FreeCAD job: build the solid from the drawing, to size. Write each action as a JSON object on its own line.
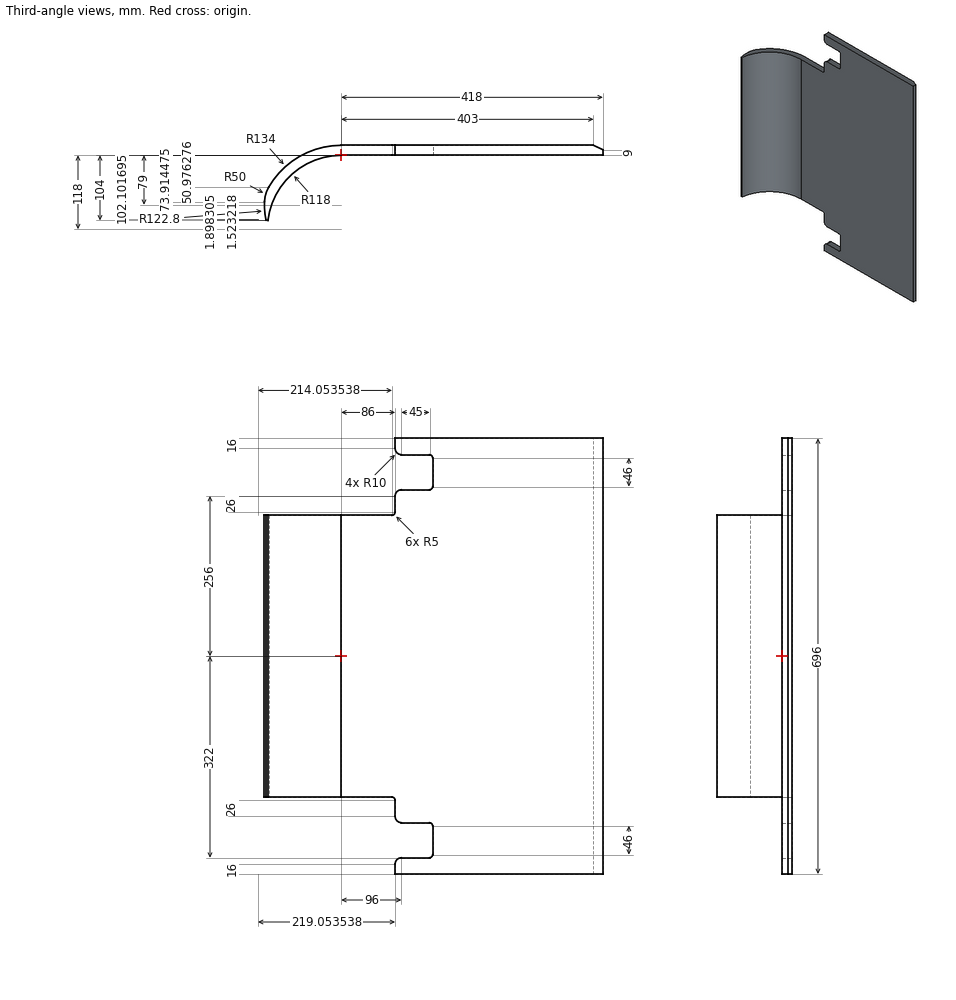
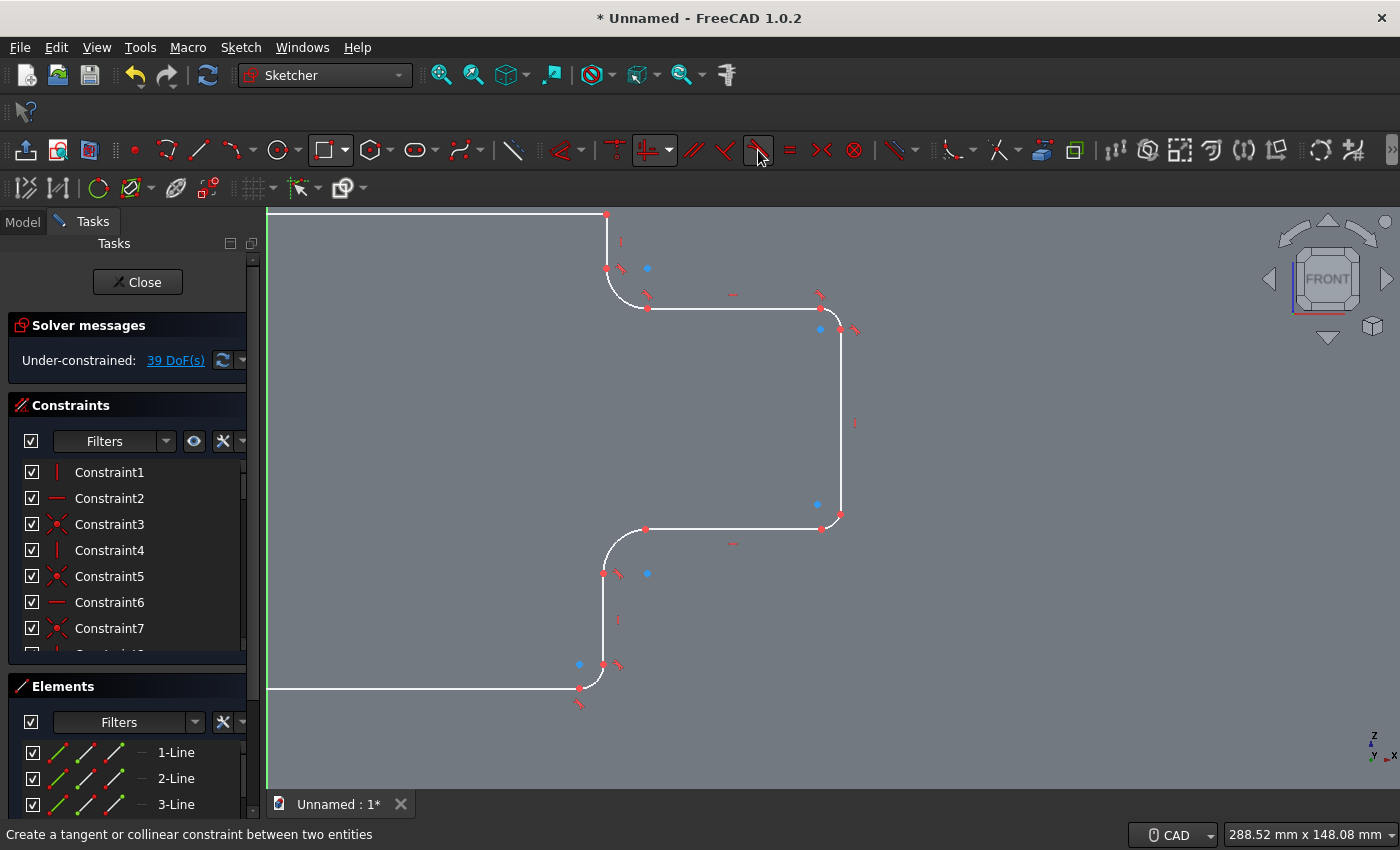
{"action": "scroll", "coordinate": [838, 330], "scroll_direction": "down", "scroll_amount": 10}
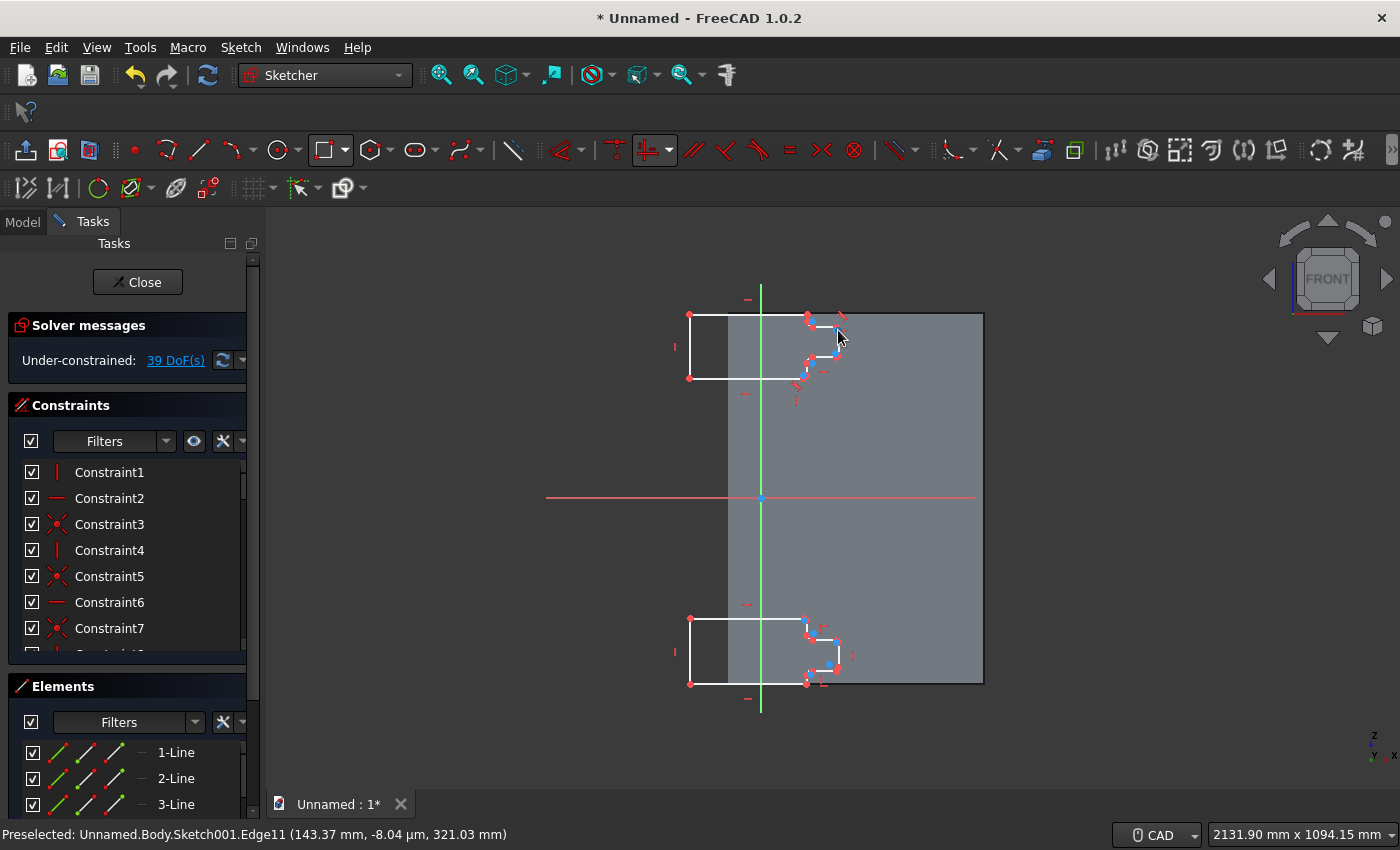
{"action": "scroll", "coordinate": [839, 338], "scroll_direction": "up", "scroll_amount": 4}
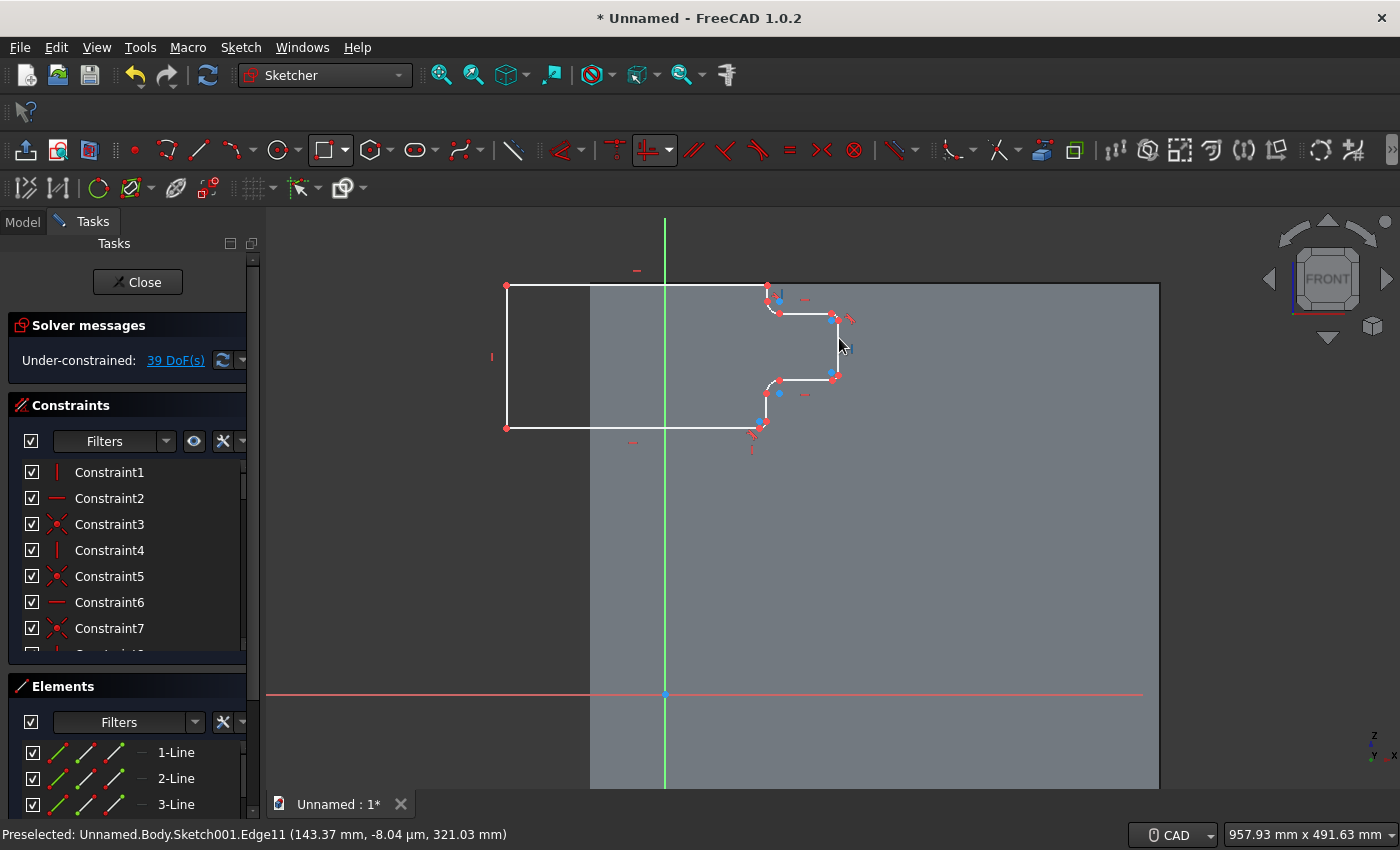
{"action": "left_click", "coordinate": [838, 337]}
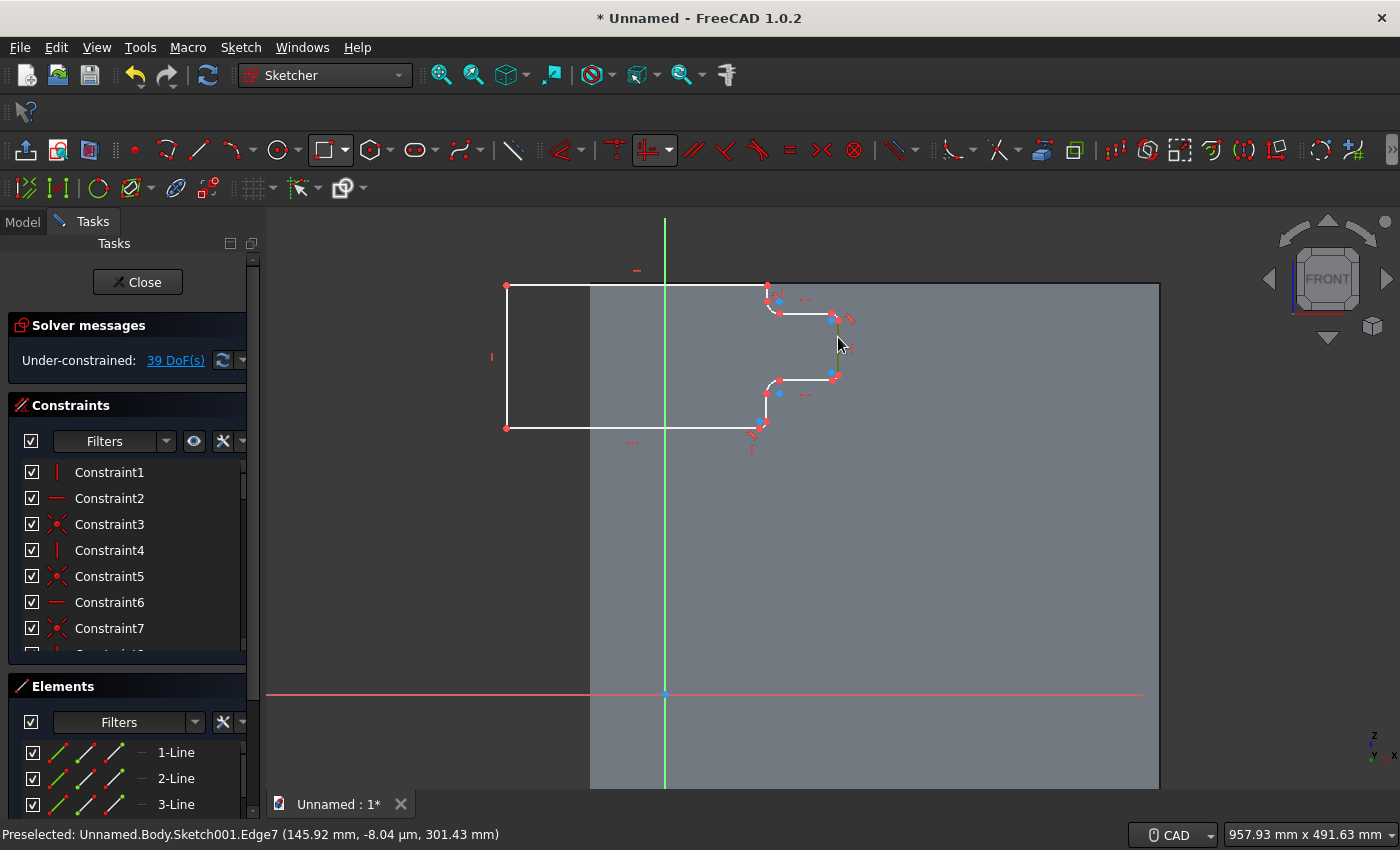
{"action": "scroll", "coordinate": [836, 379], "scroll_direction": "up", "scroll_amount": 7}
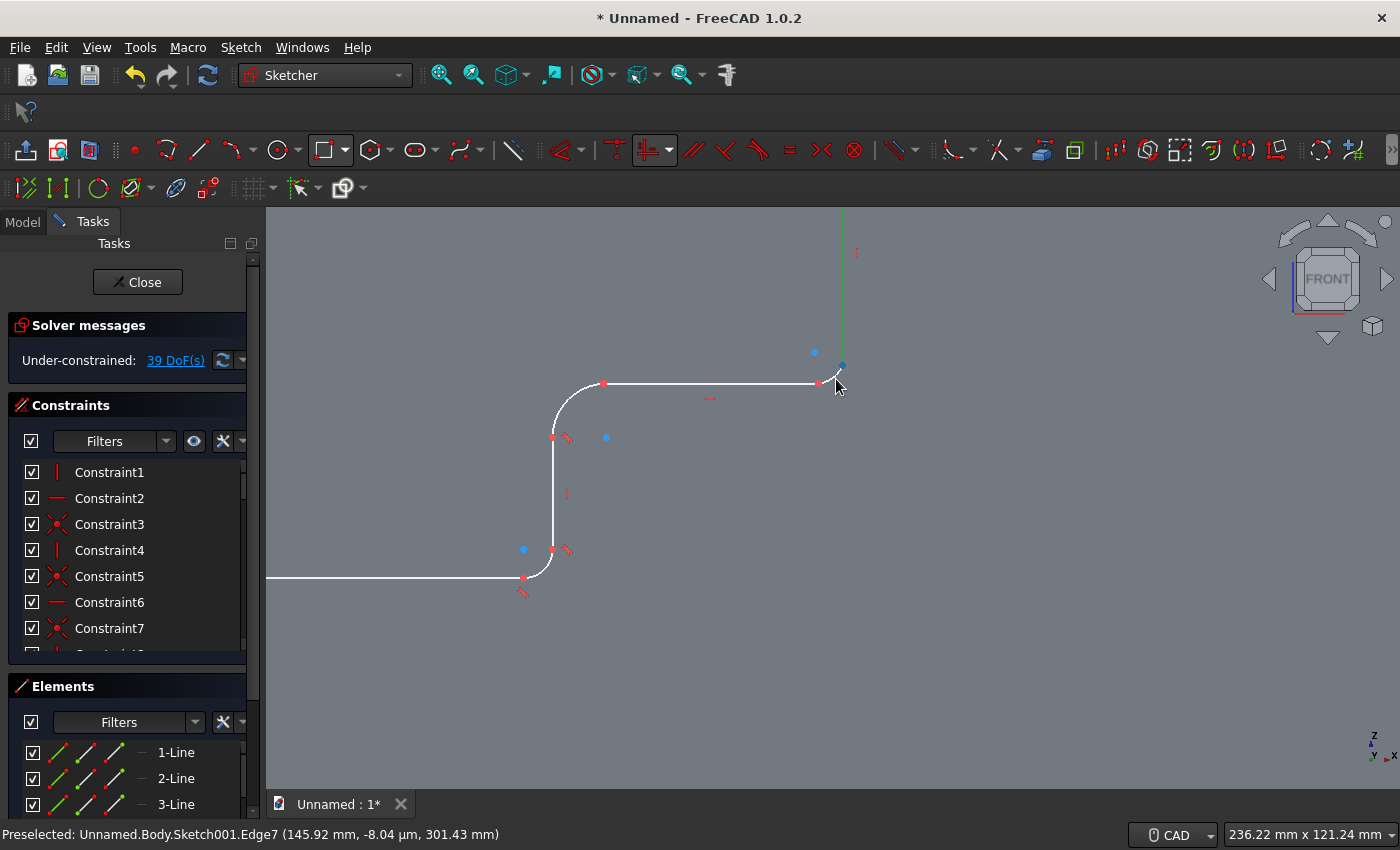
{"action": "left_click", "coordinate": [833, 378]}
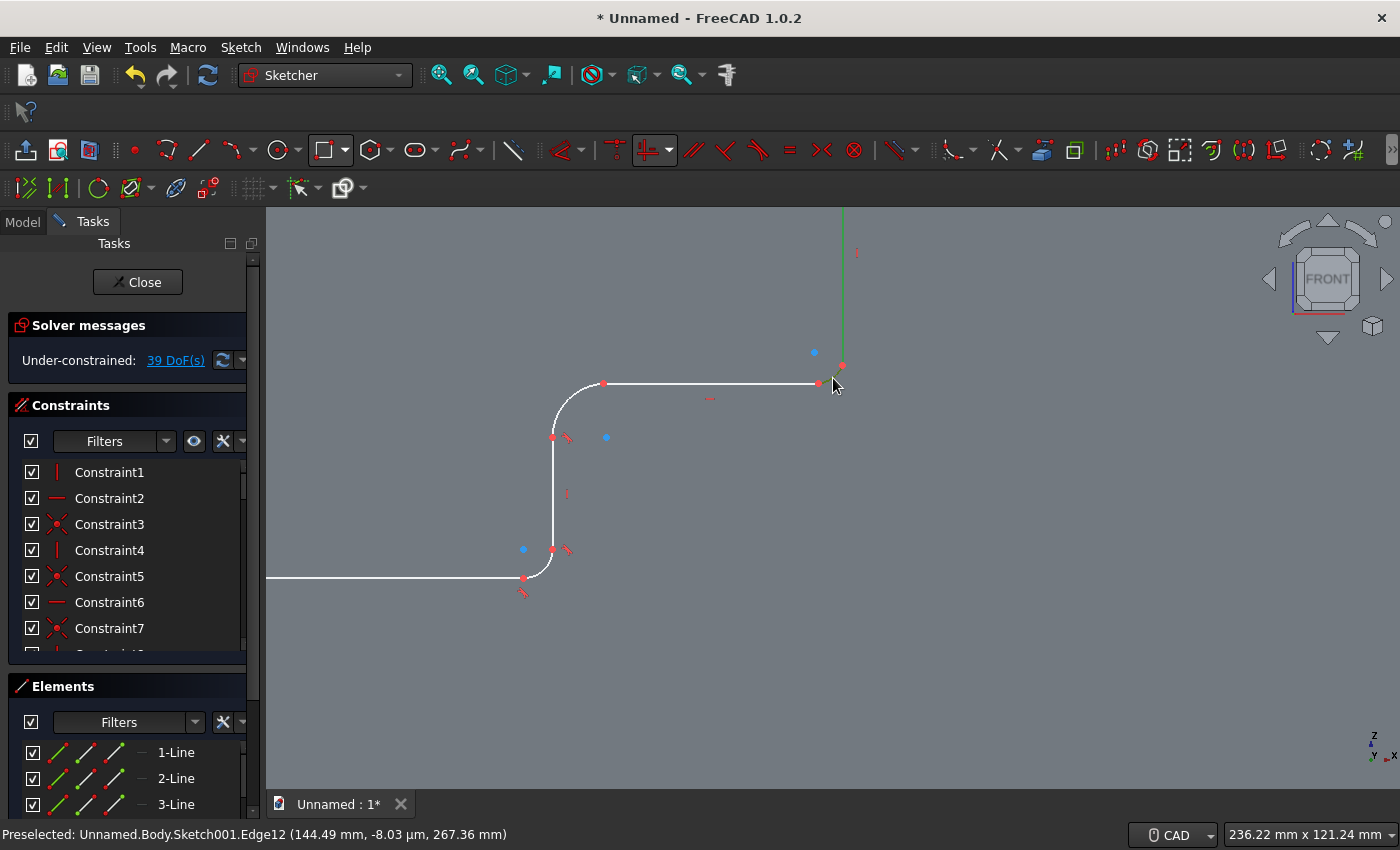
{"action": "left_click", "coordinate": [758, 150]}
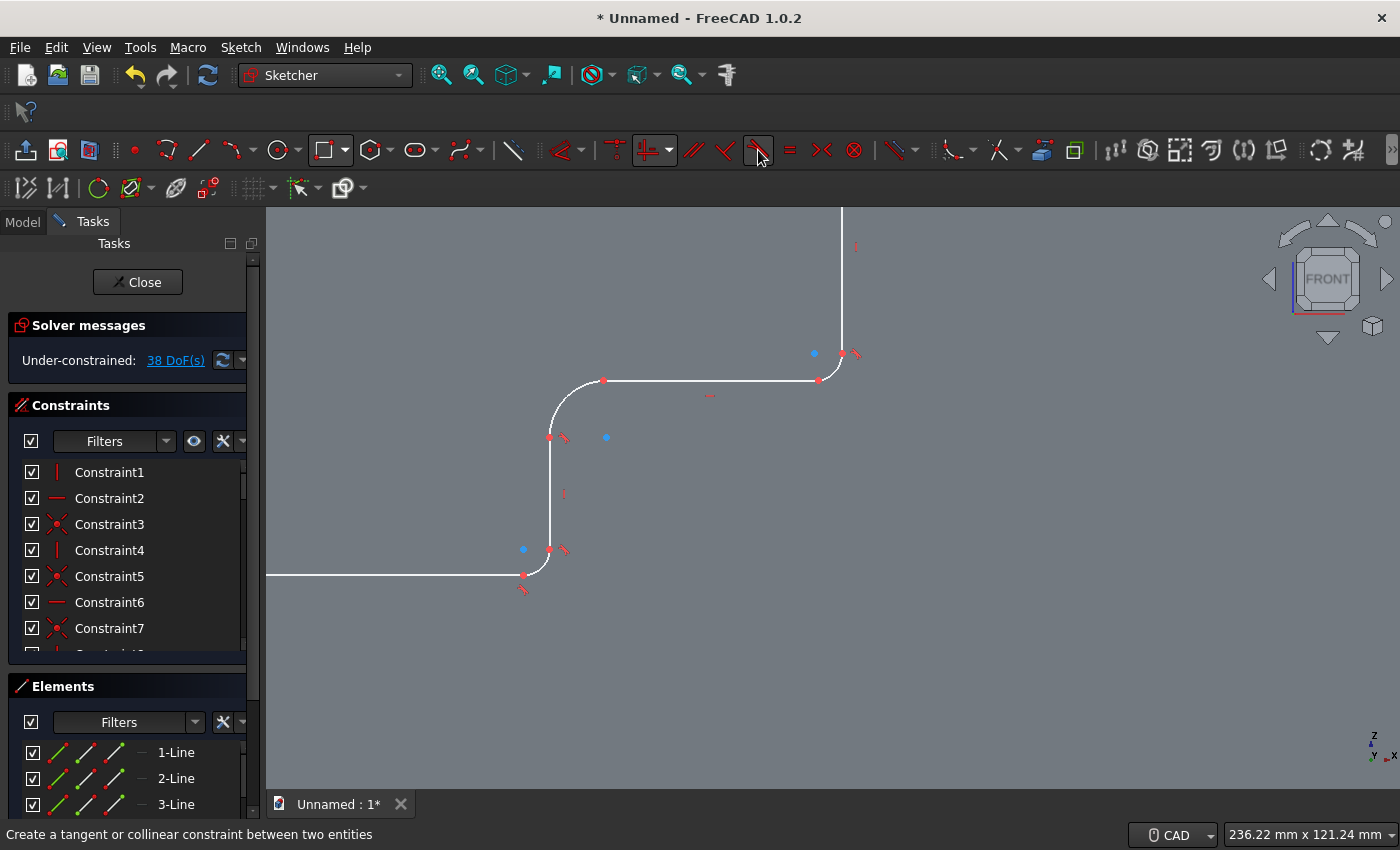
{"action": "scroll", "coordinate": [838, 353], "scroll_direction": "down", "scroll_amount": 11}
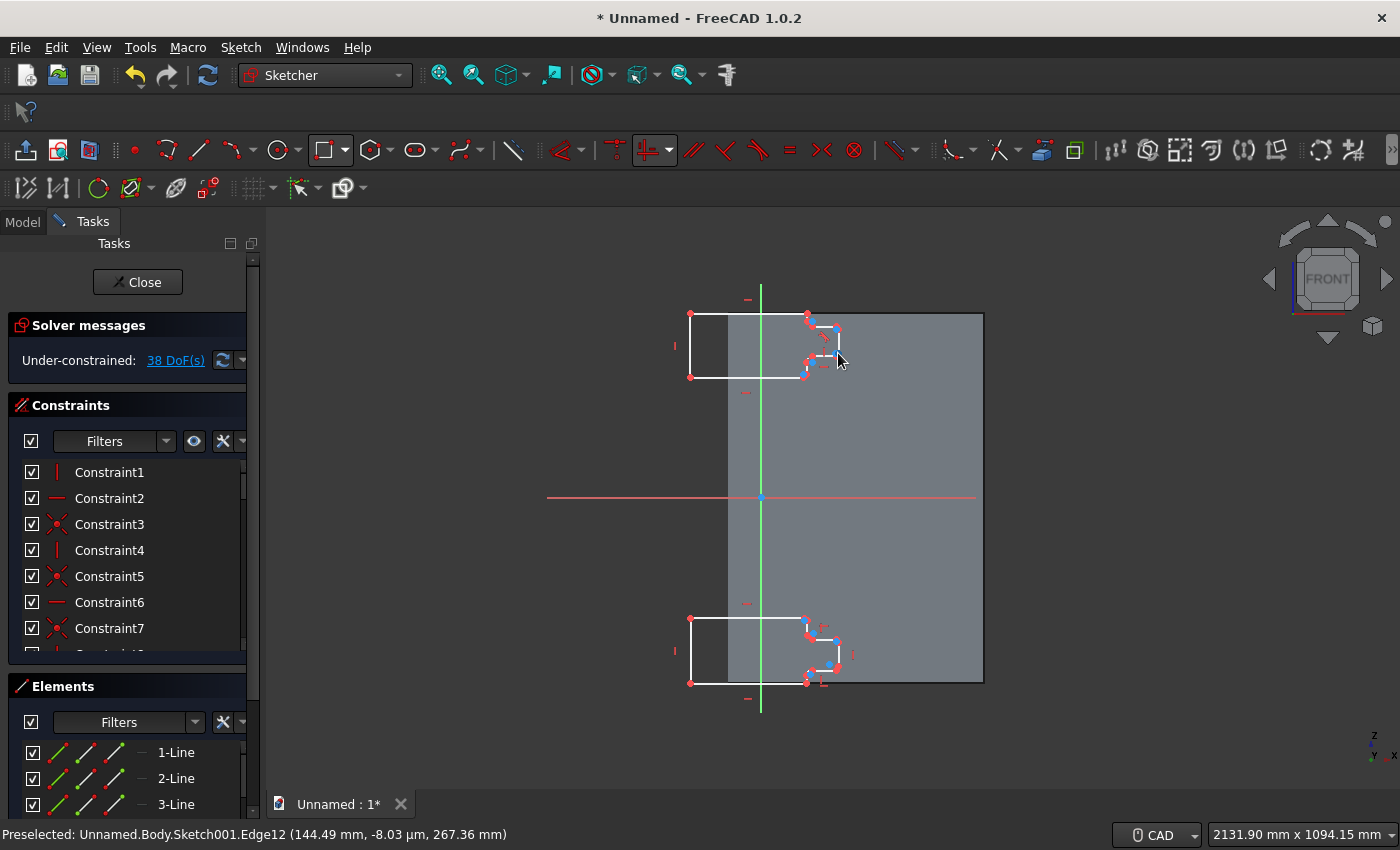
{"action": "scroll", "coordinate": [829, 356], "scroll_direction": "up", "scroll_amount": 4}